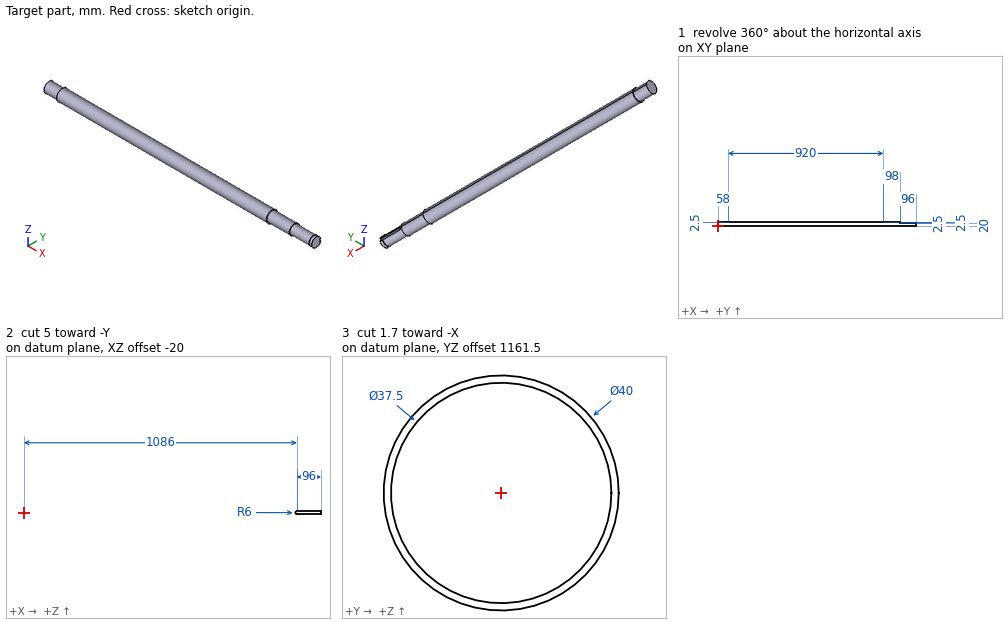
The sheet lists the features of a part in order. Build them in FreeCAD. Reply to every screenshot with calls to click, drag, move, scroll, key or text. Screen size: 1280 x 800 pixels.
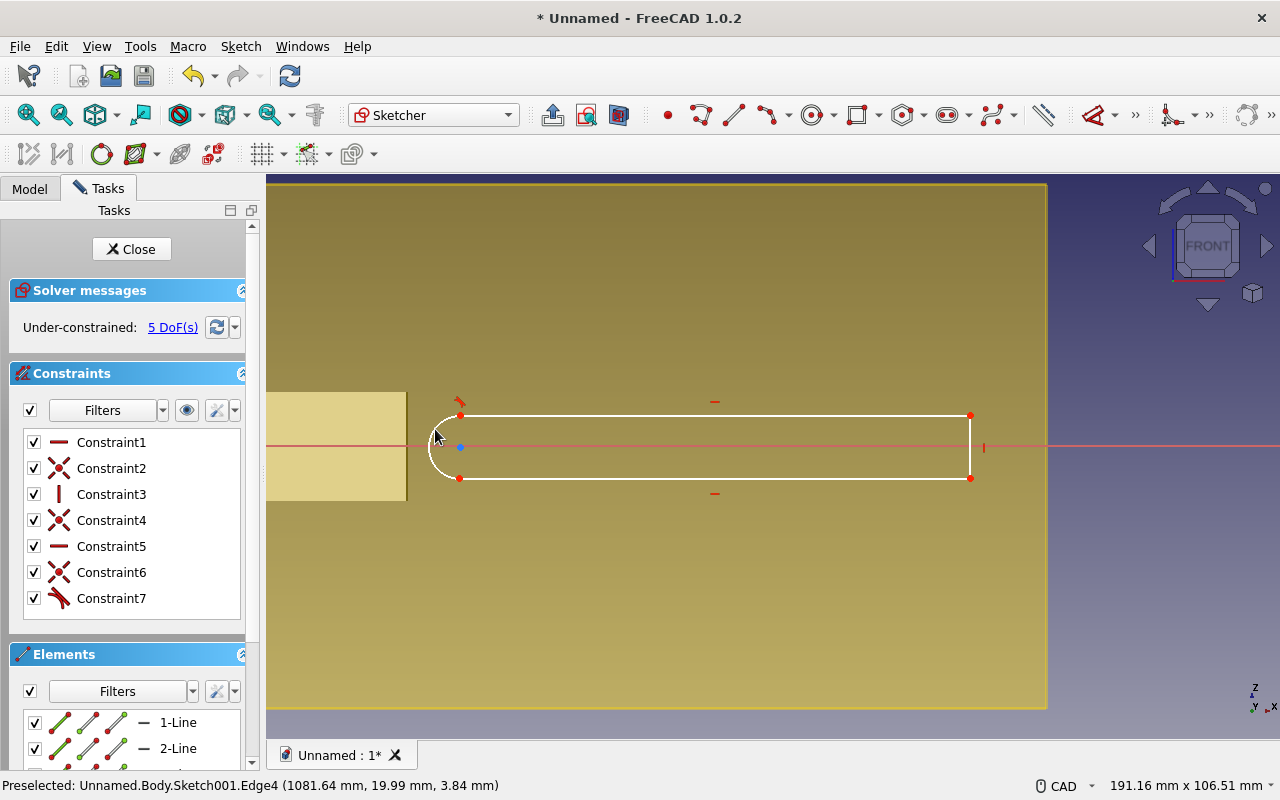
click(817, 479)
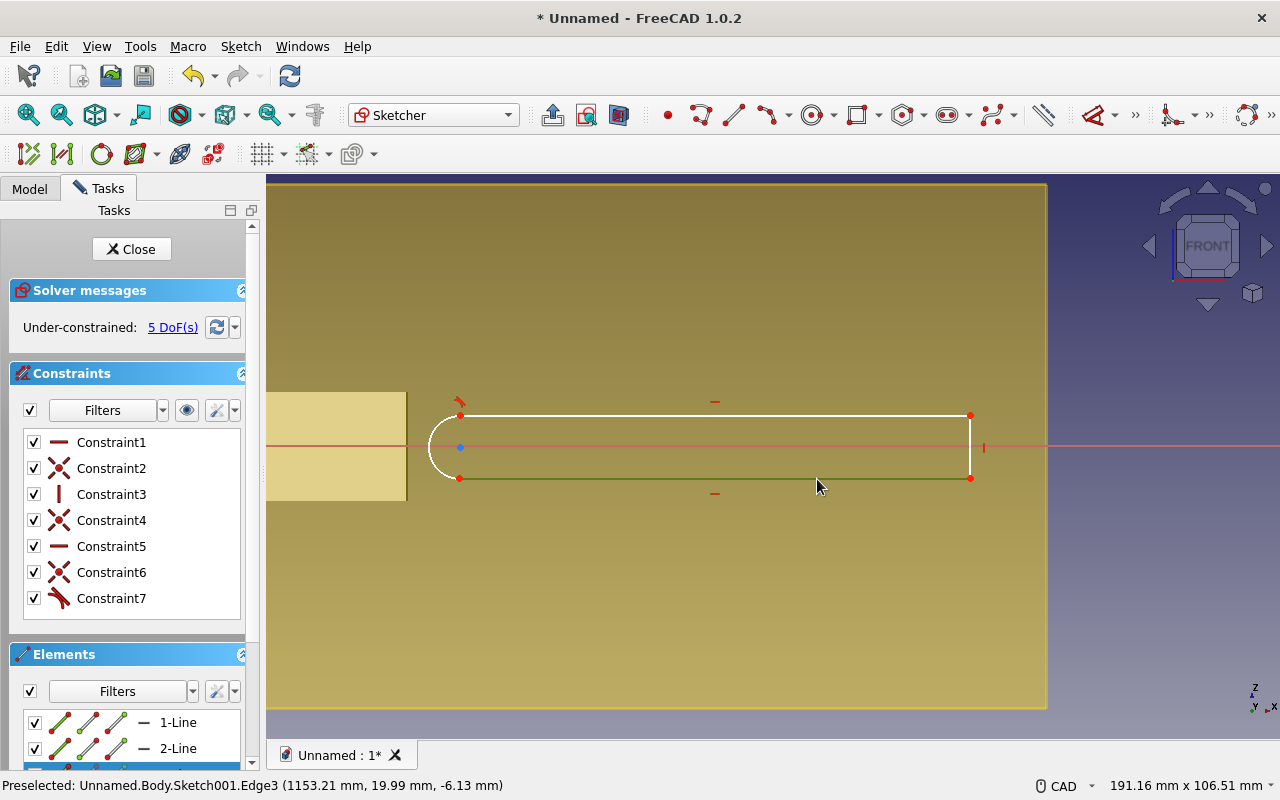
click(435, 429)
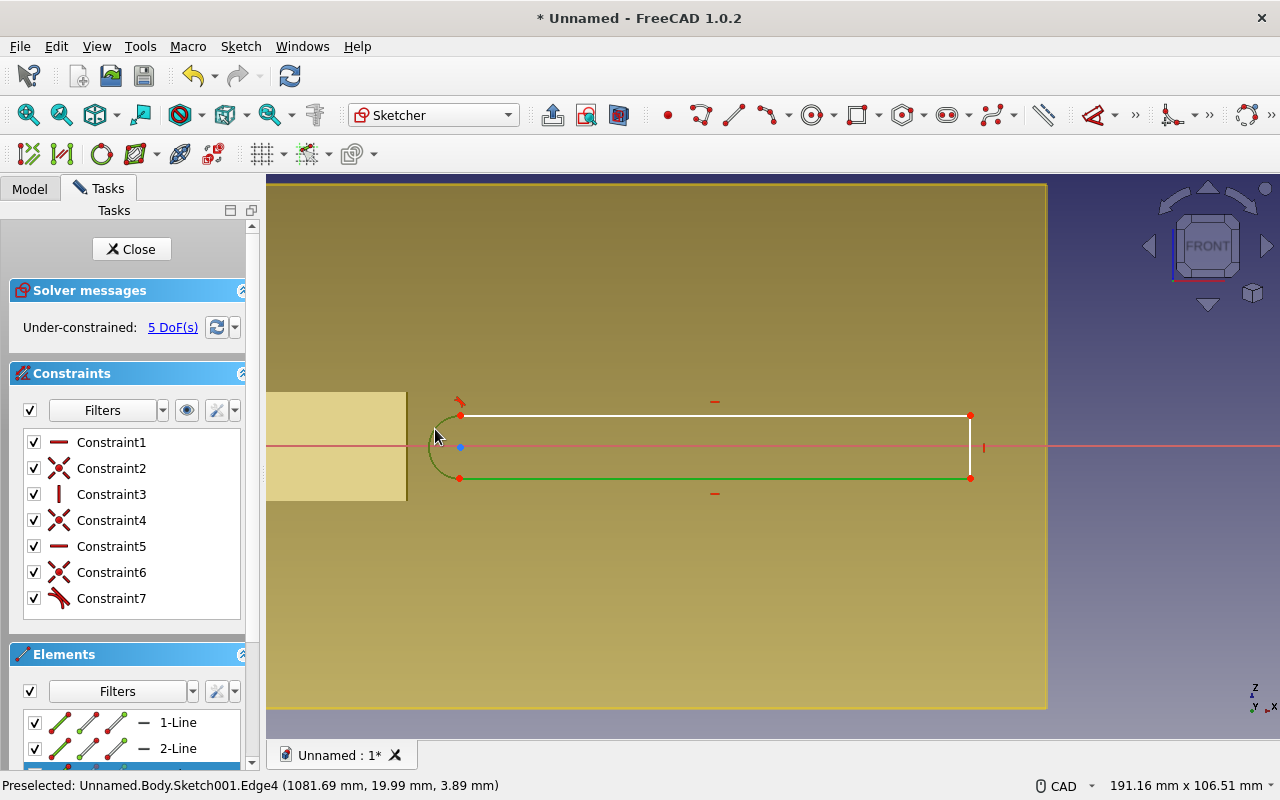
key(t)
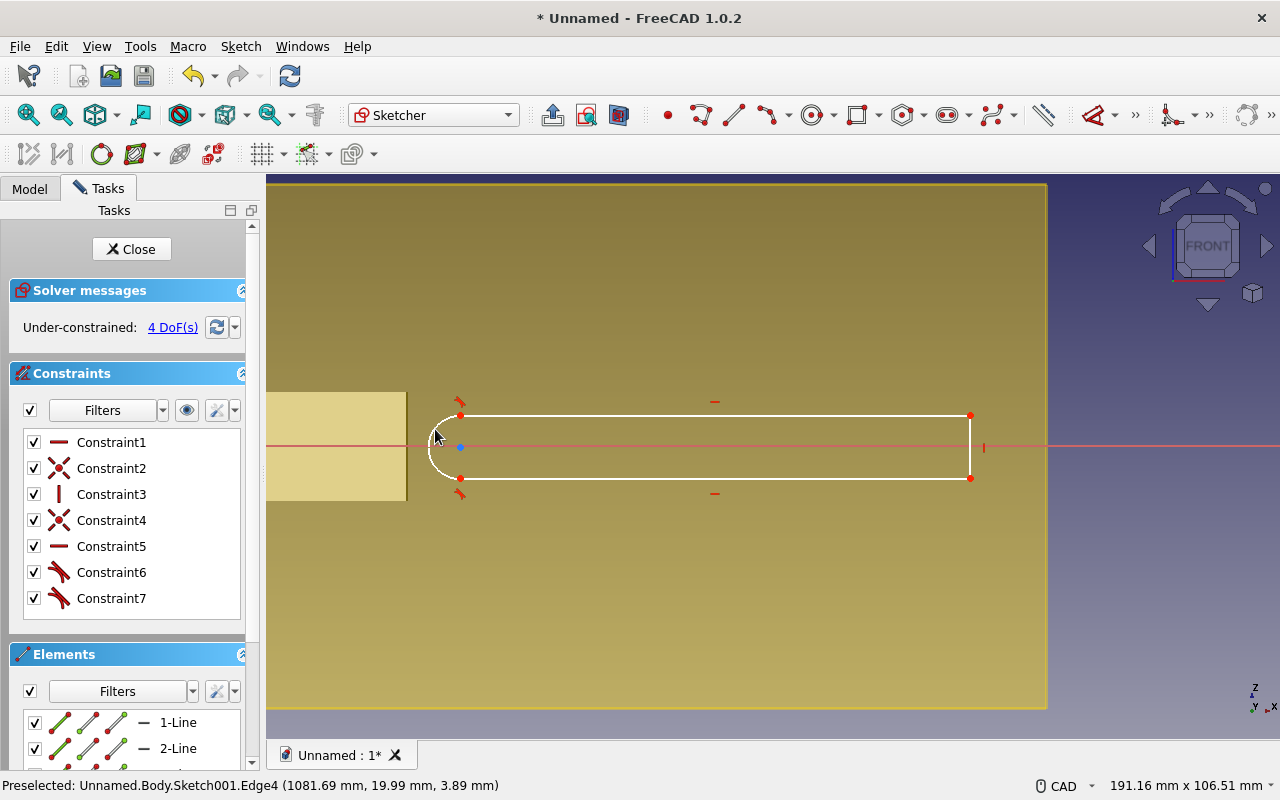
click(460, 447)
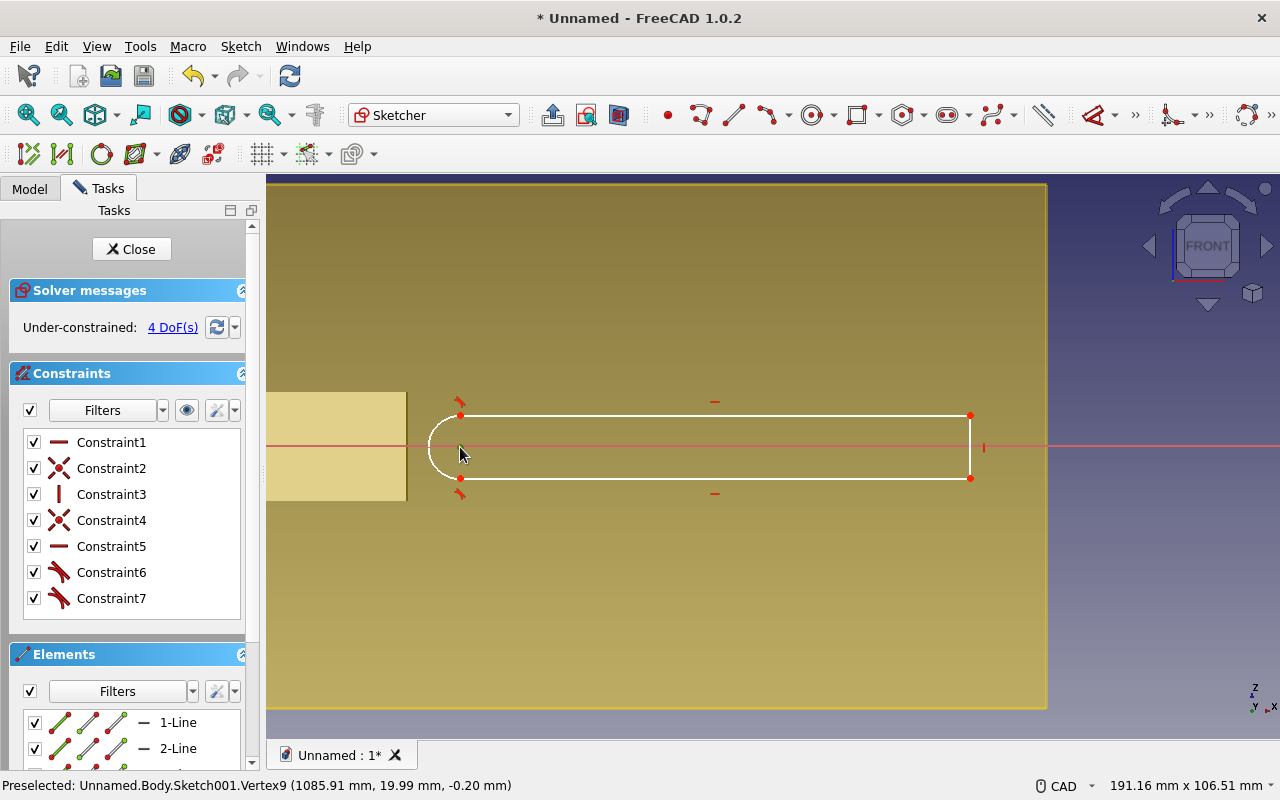
click(353, 446)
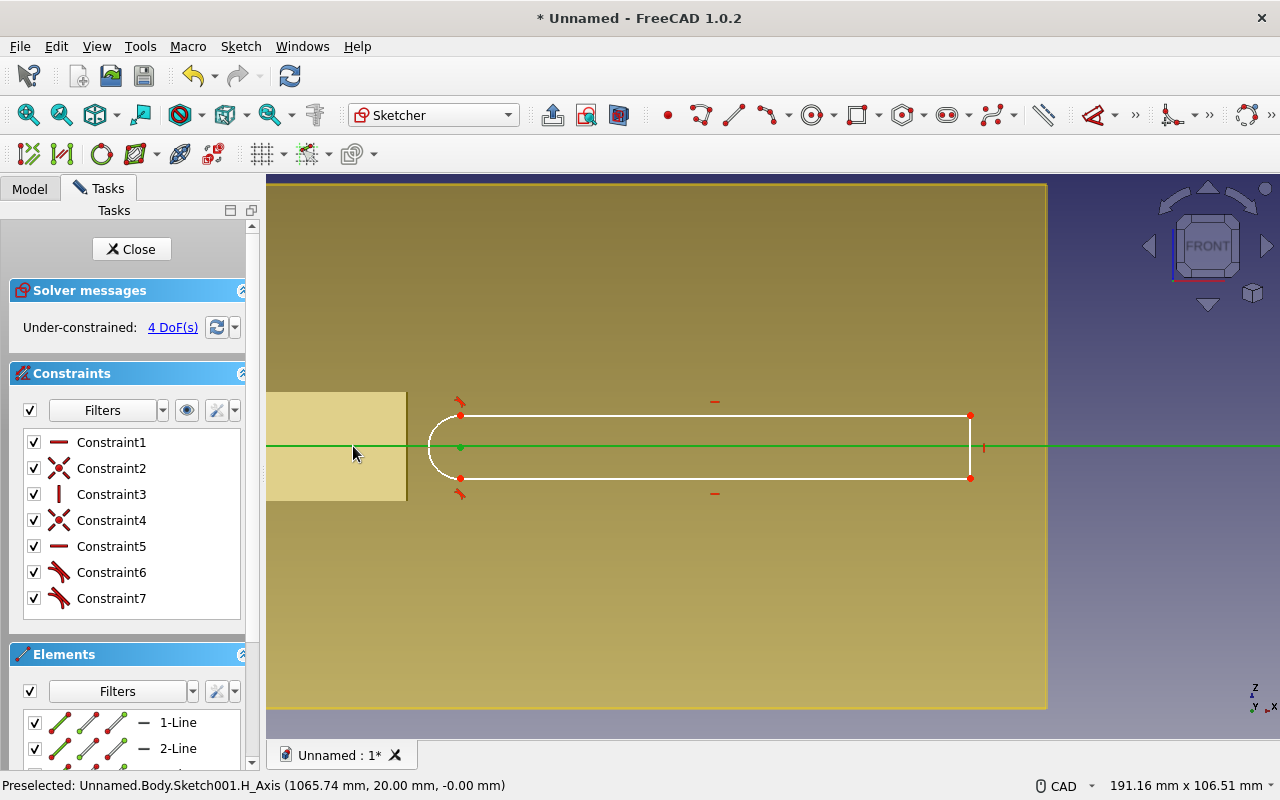
key(c)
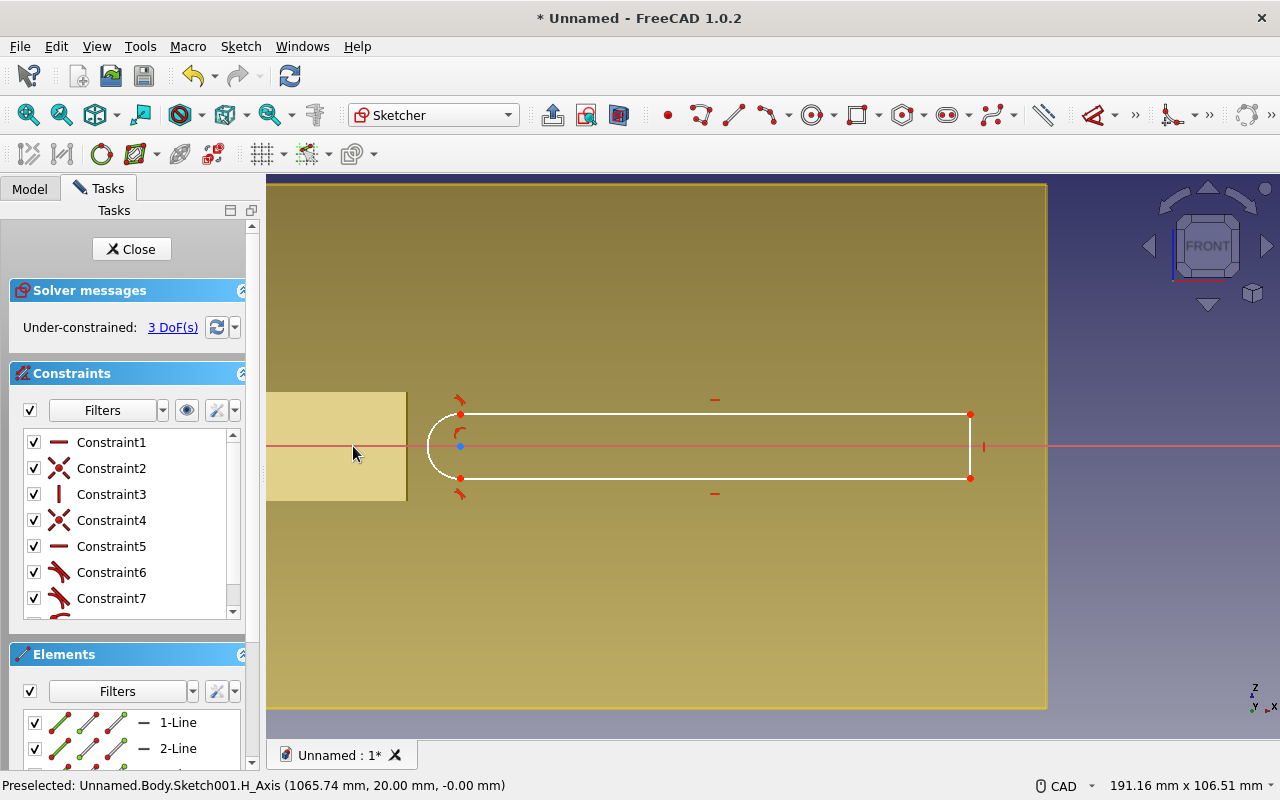
click(1092, 116)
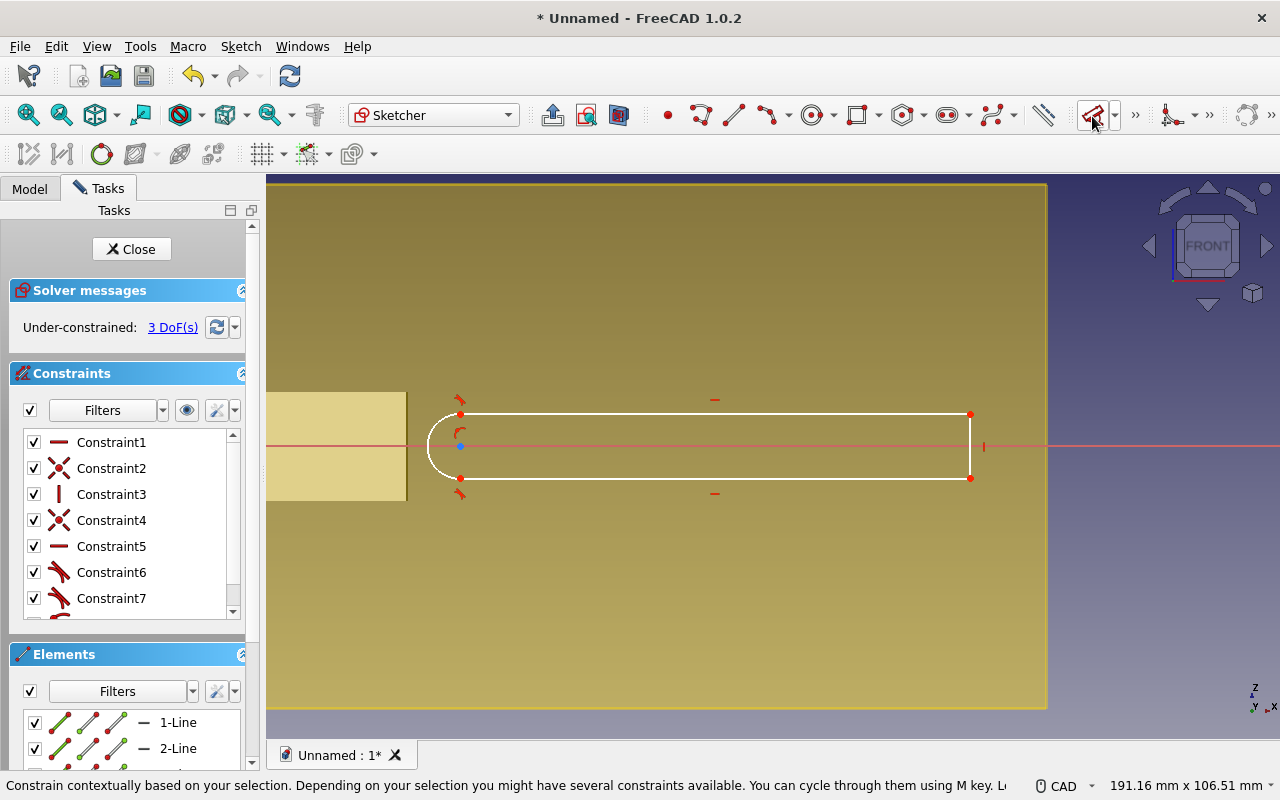
scroll(434, 427, up, 2)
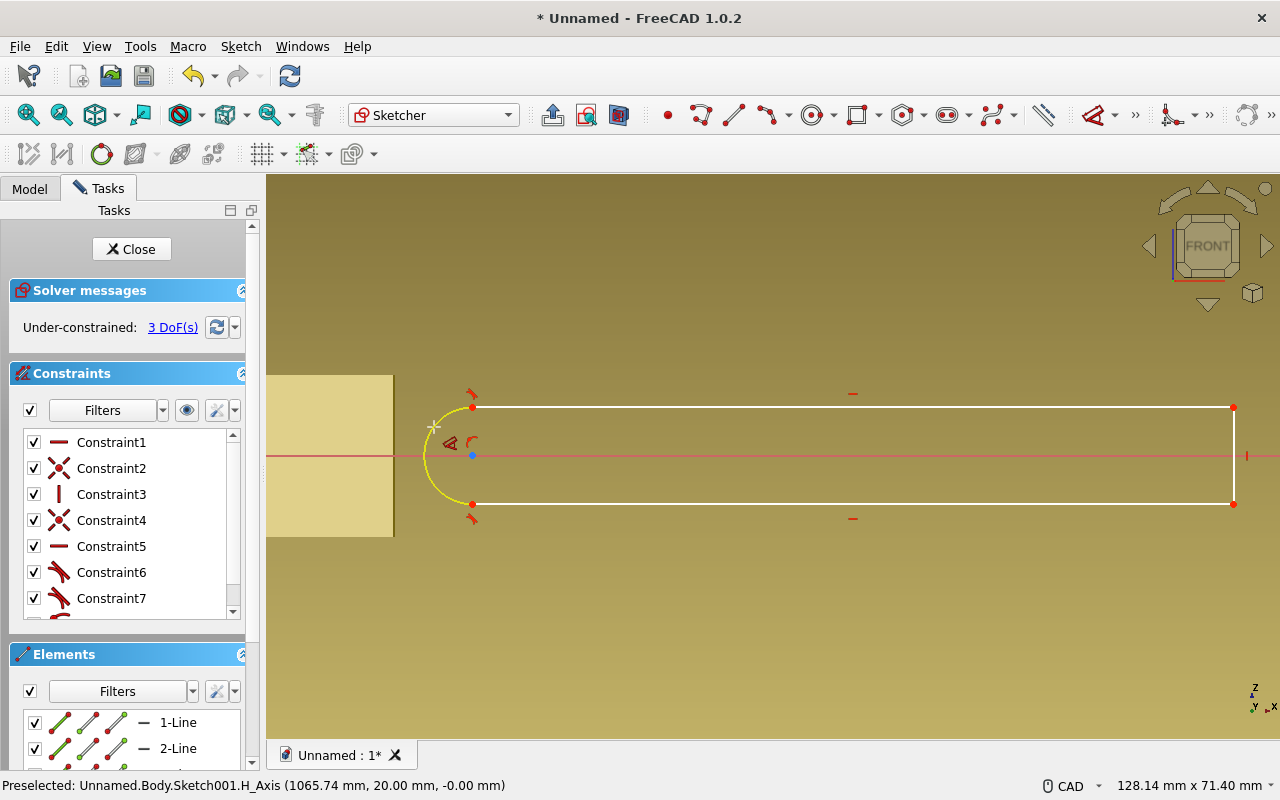
click(434, 427)
click(408, 408)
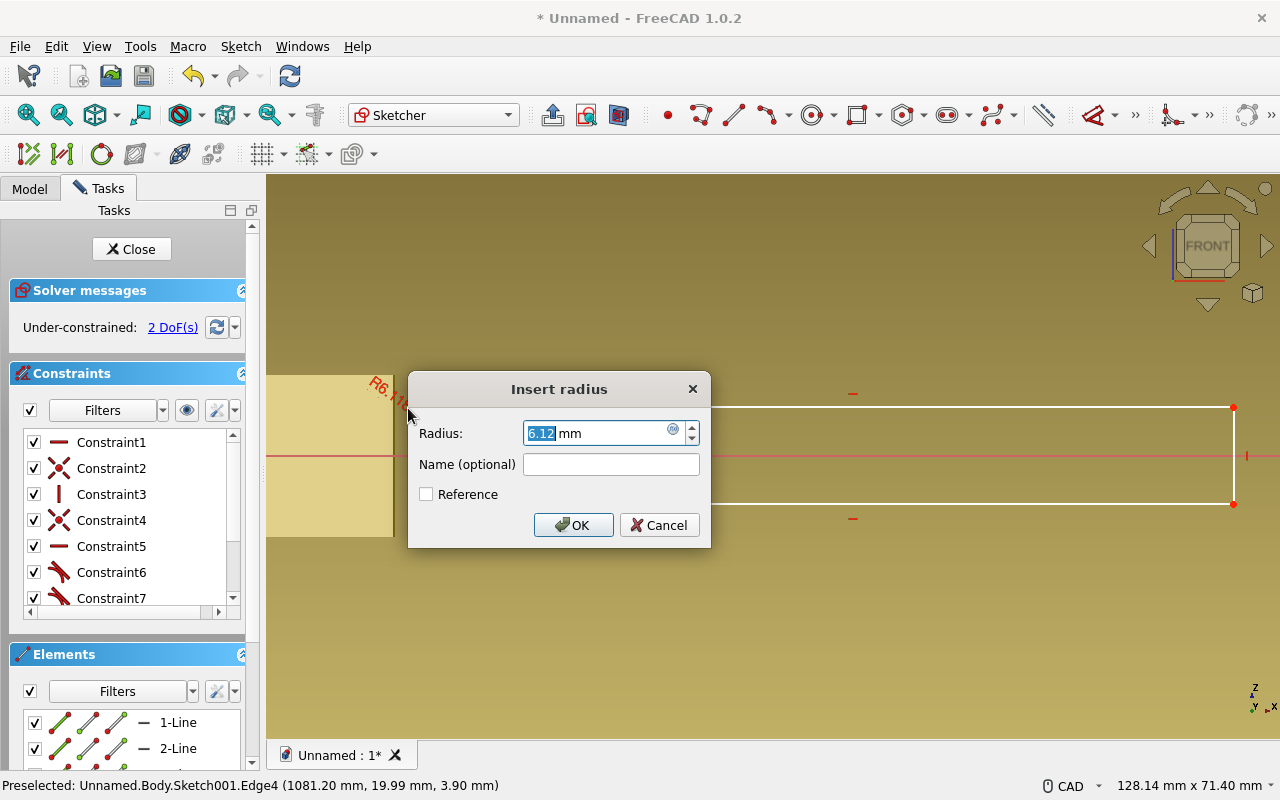
text(6)
key(Return)